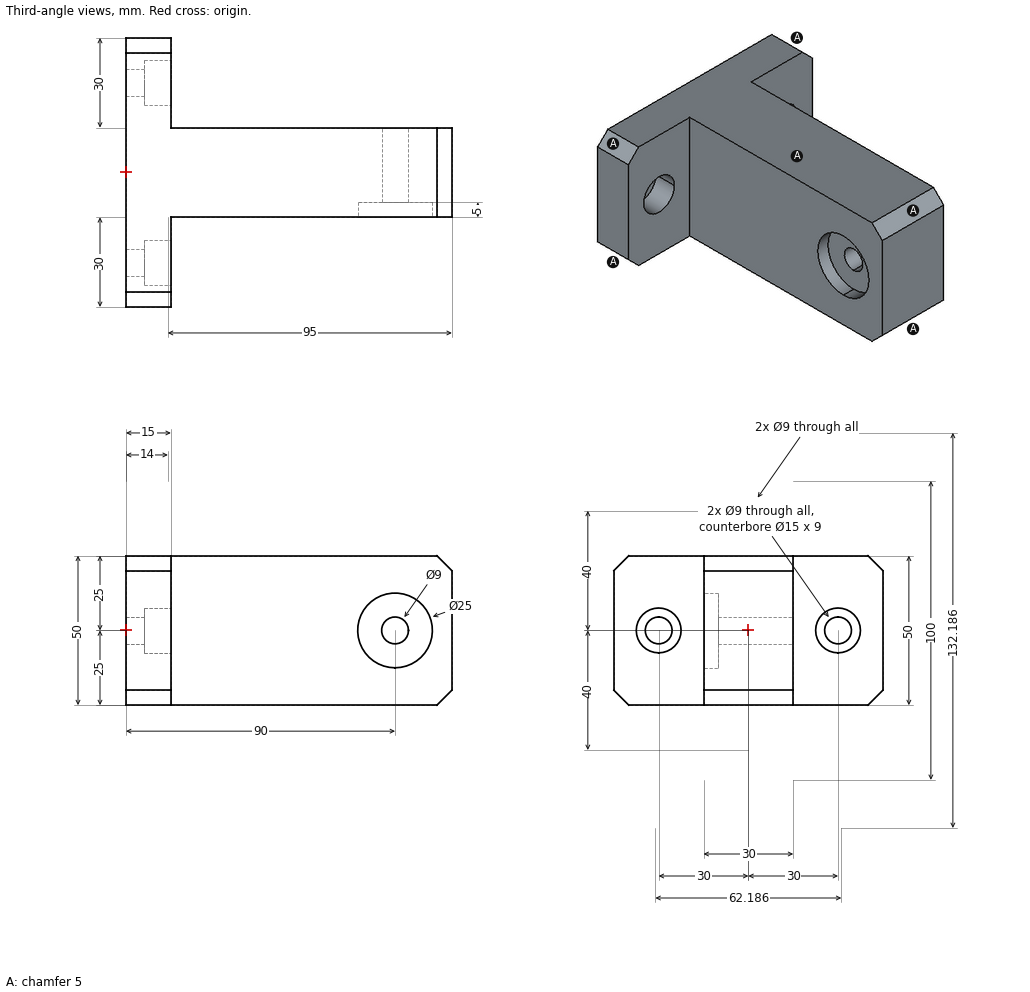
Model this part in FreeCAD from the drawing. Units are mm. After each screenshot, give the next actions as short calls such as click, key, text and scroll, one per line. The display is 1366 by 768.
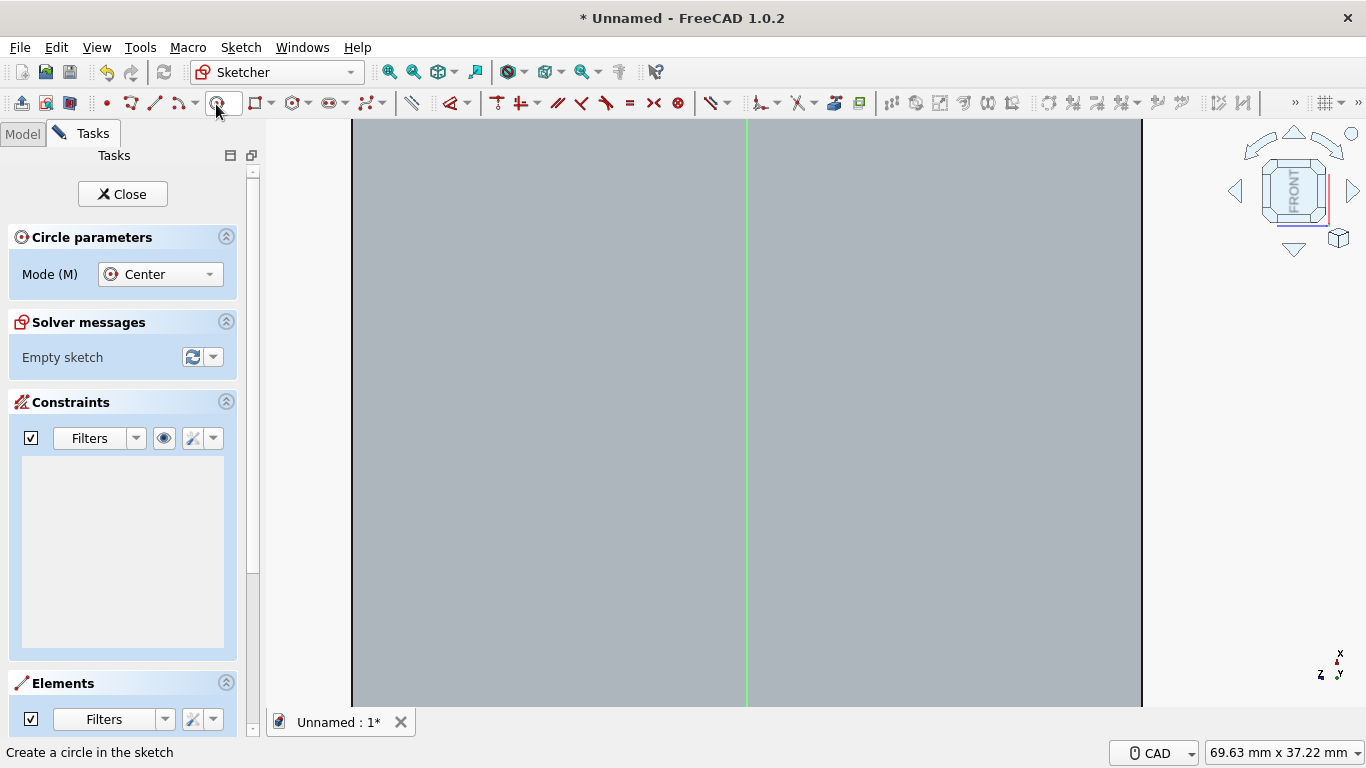
click(747, 414)
move(887, 274)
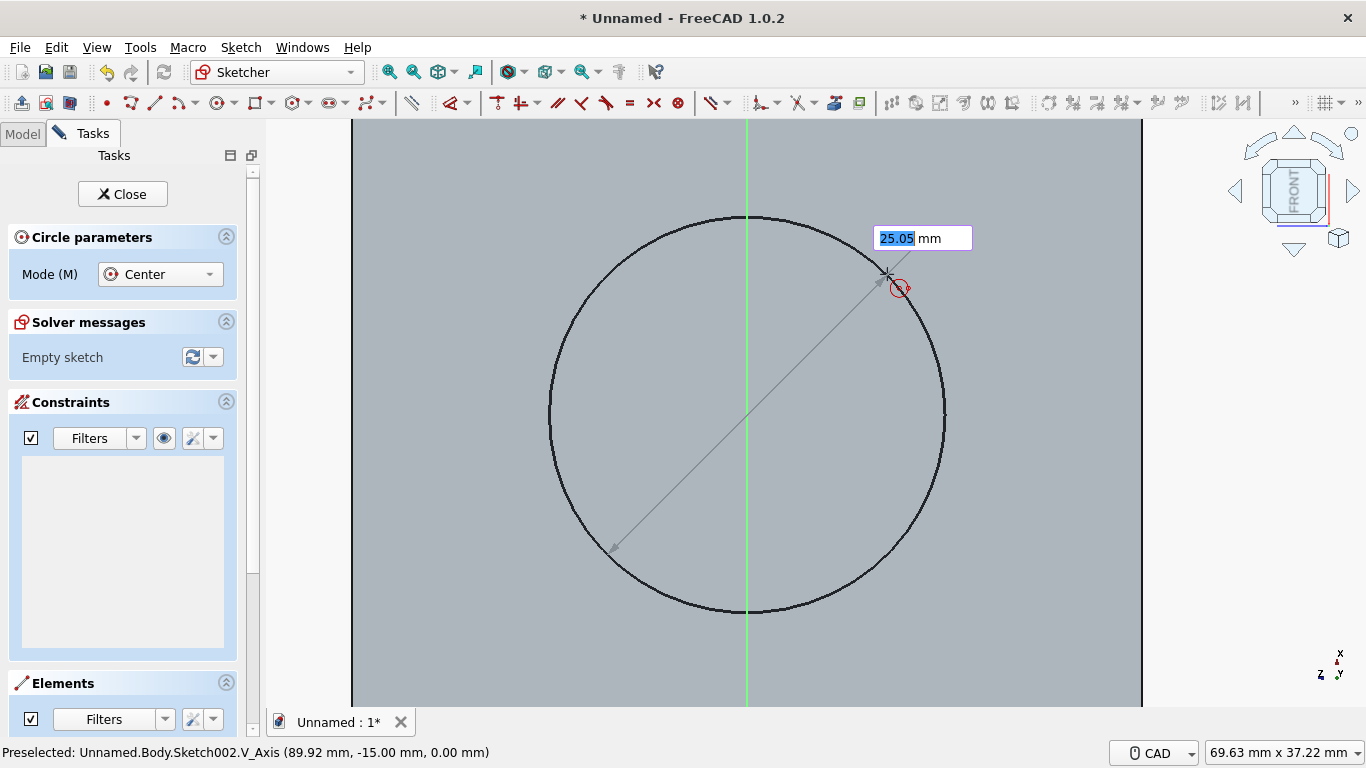
text(25)
key(Return)
key(Escape)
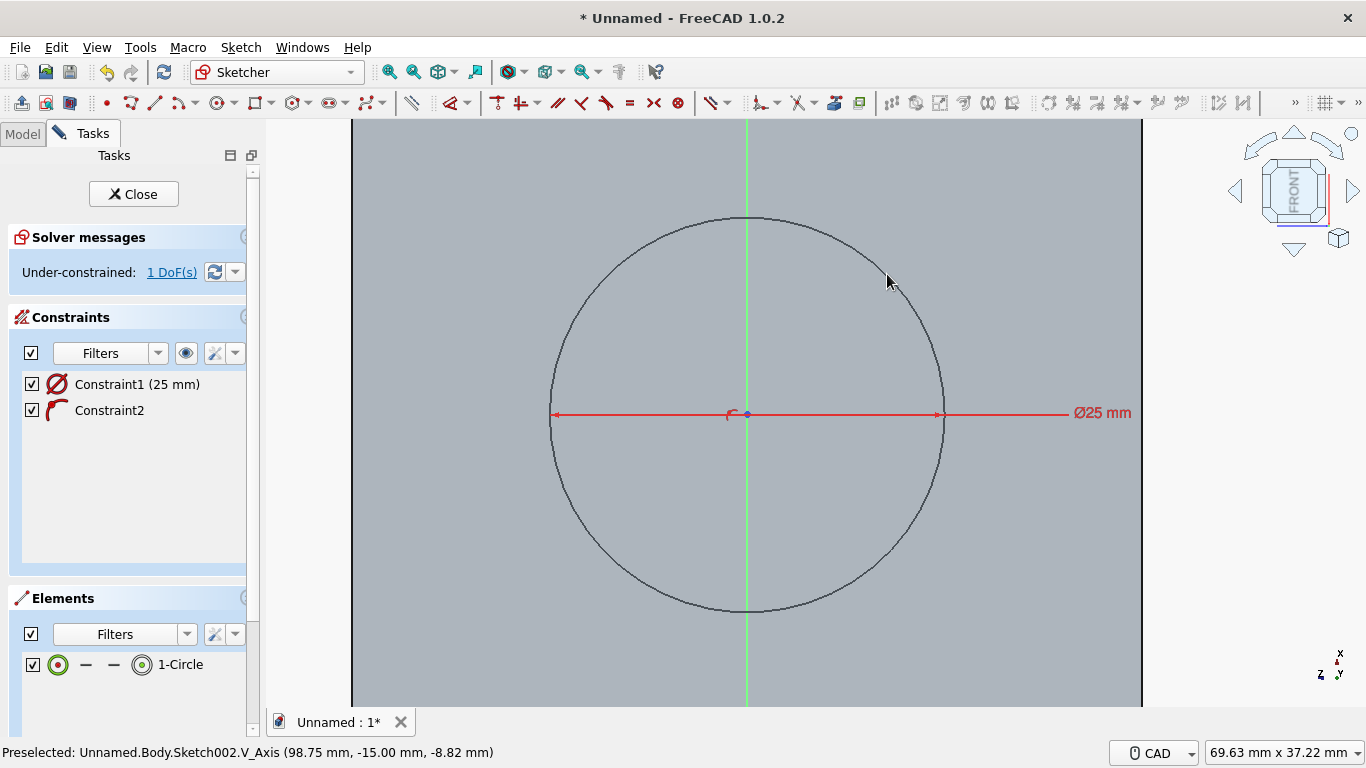
key(d)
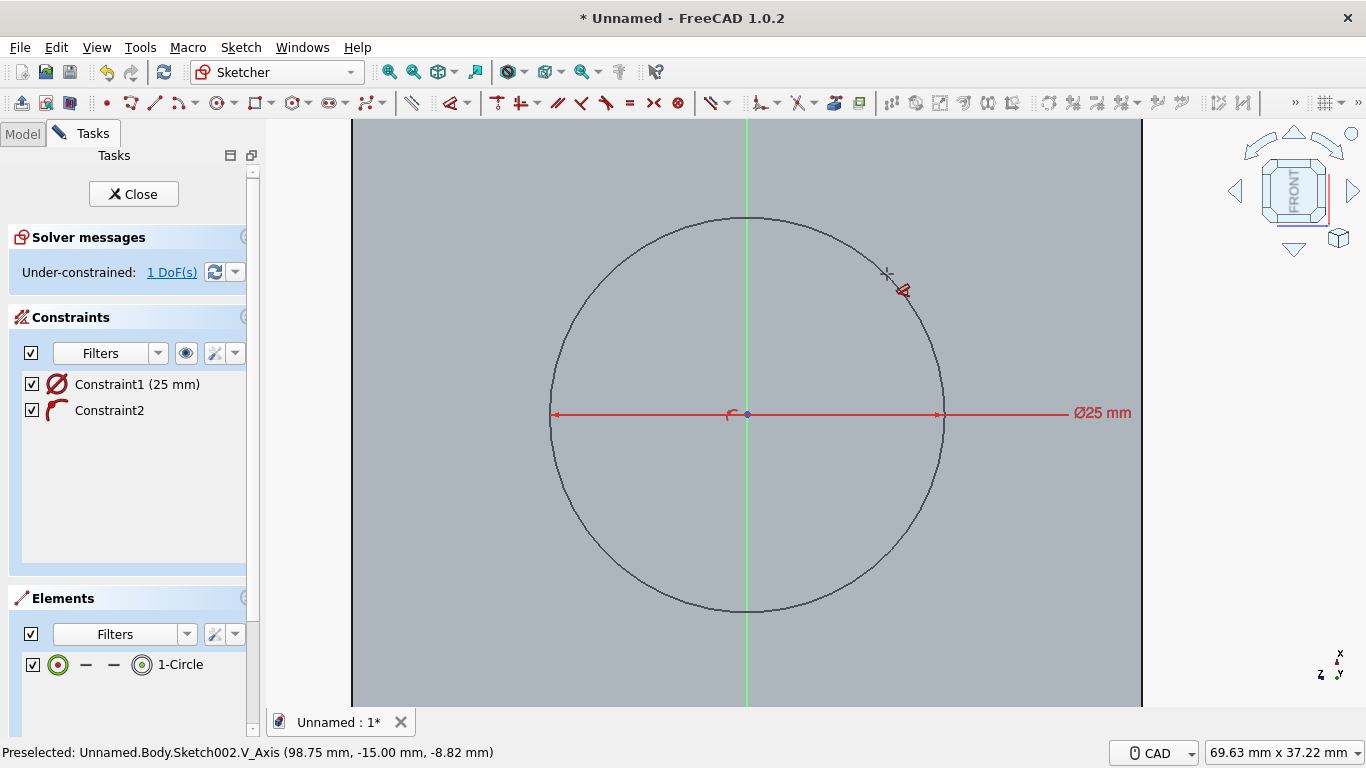
click(747, 415)
click(781, 547)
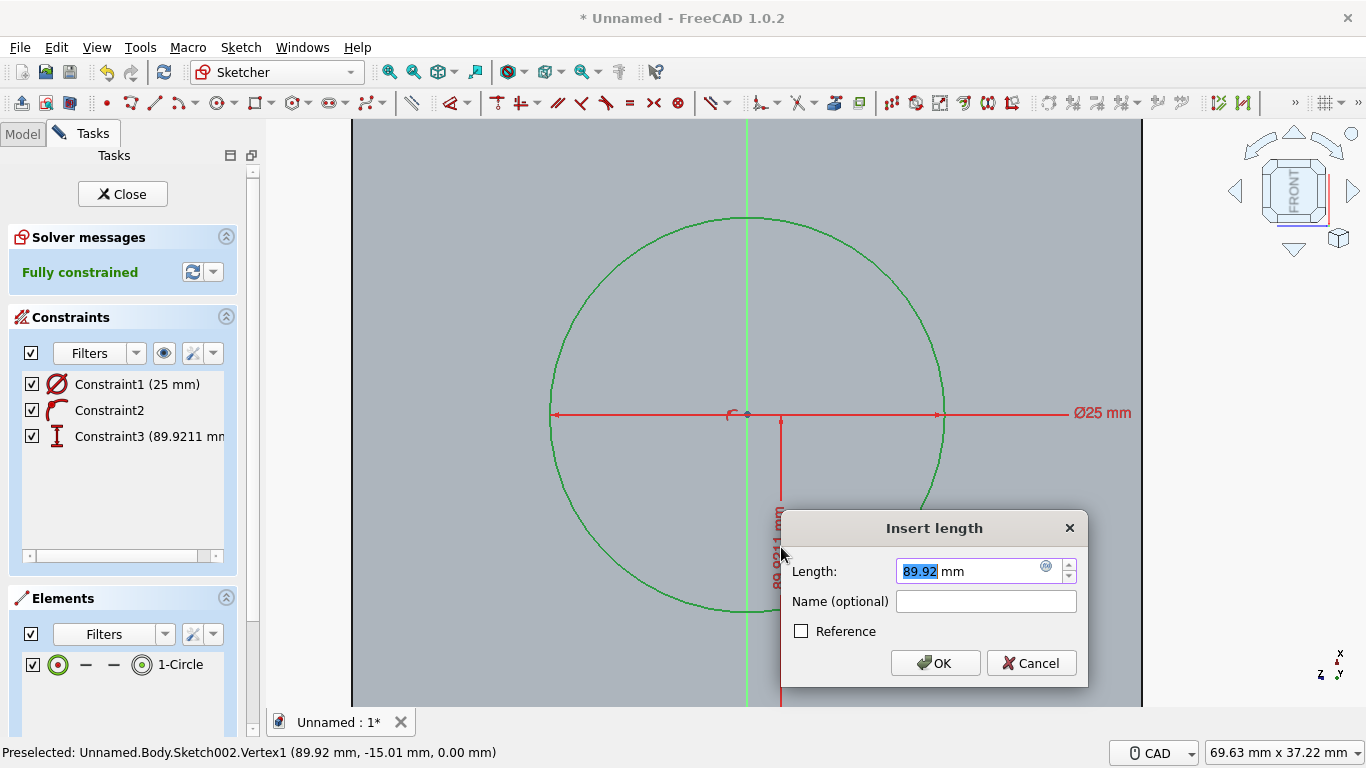
text(90)
key(Return)
key(Escape)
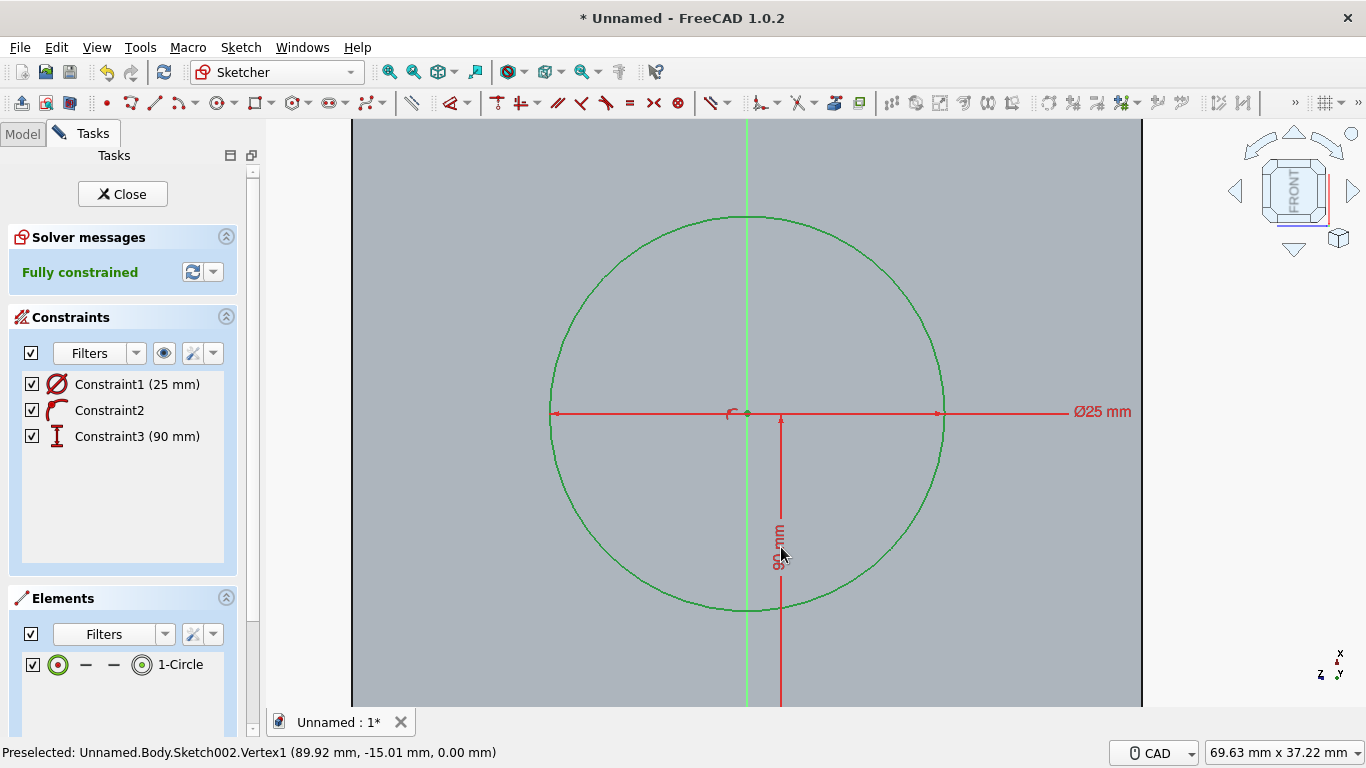
click(123, 194)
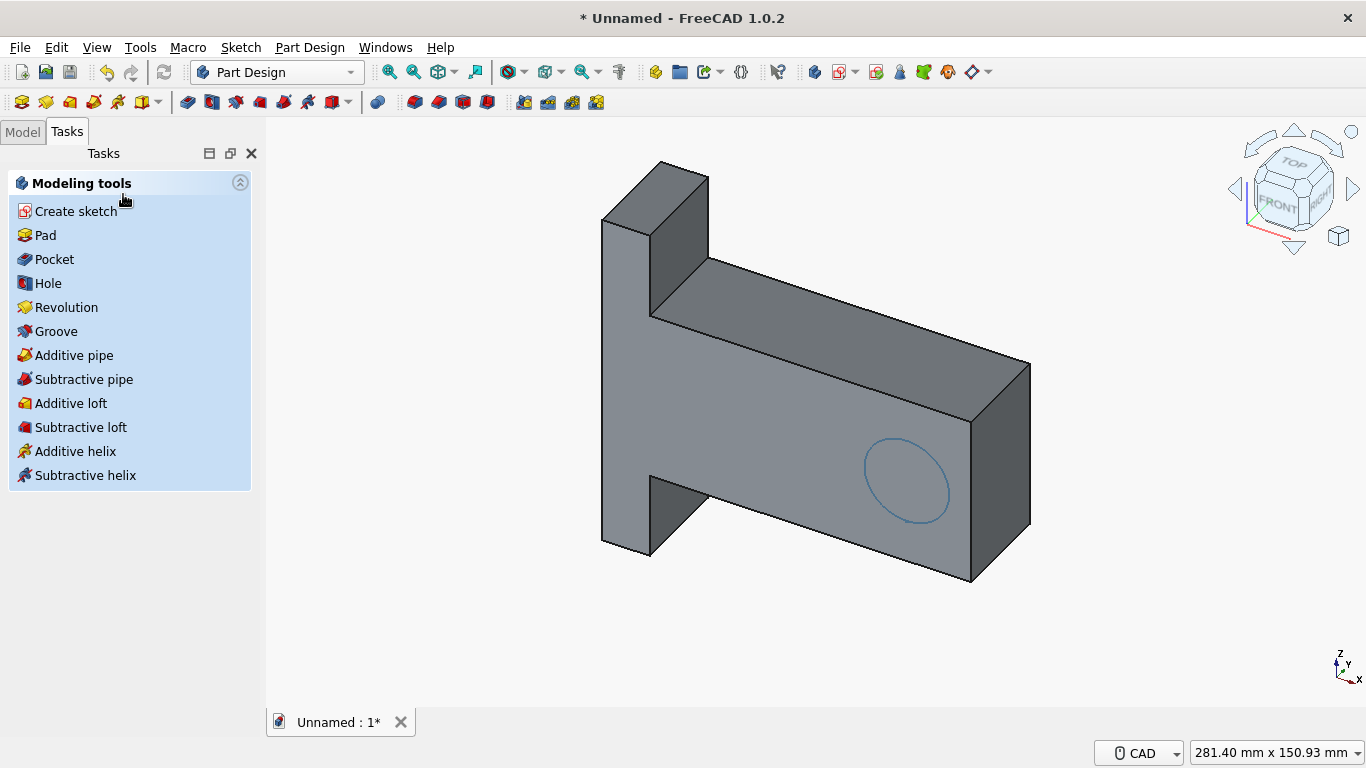
click(188, 102)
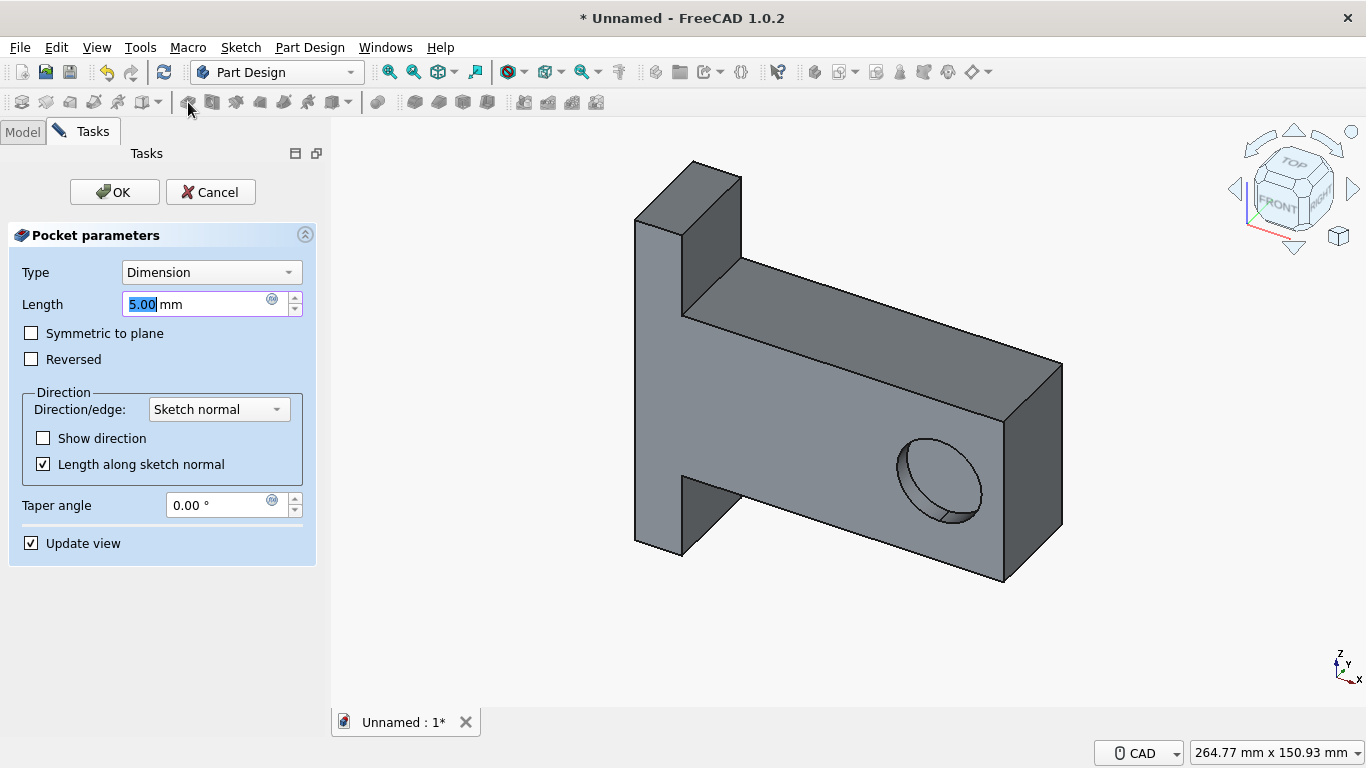
text(5)
key(Tab)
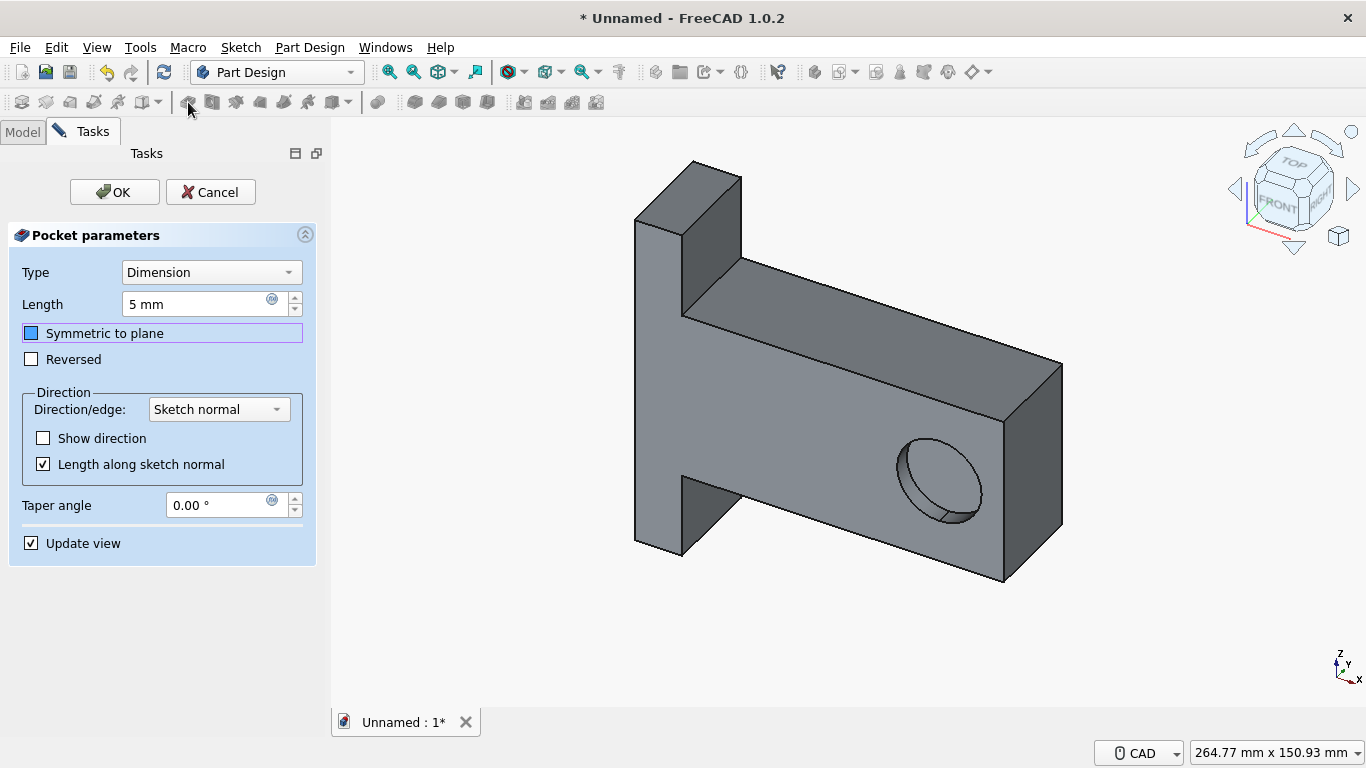
click(115, 192)